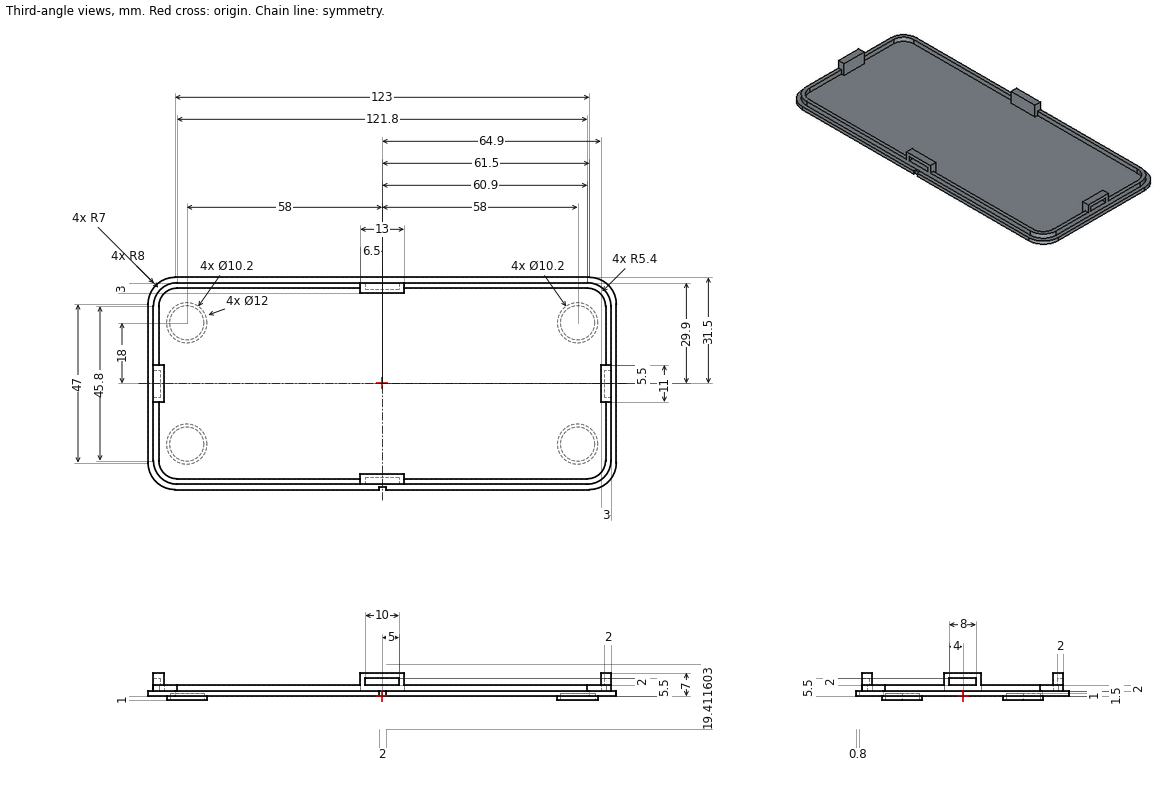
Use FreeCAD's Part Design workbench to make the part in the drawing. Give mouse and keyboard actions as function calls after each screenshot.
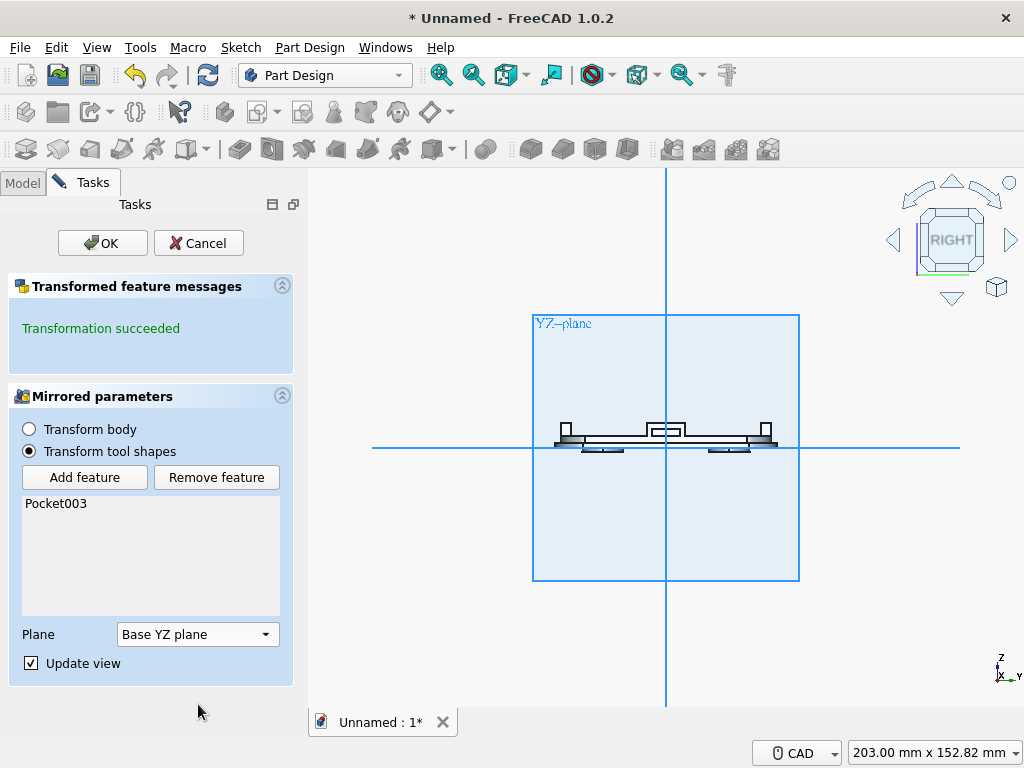
click(103, 243)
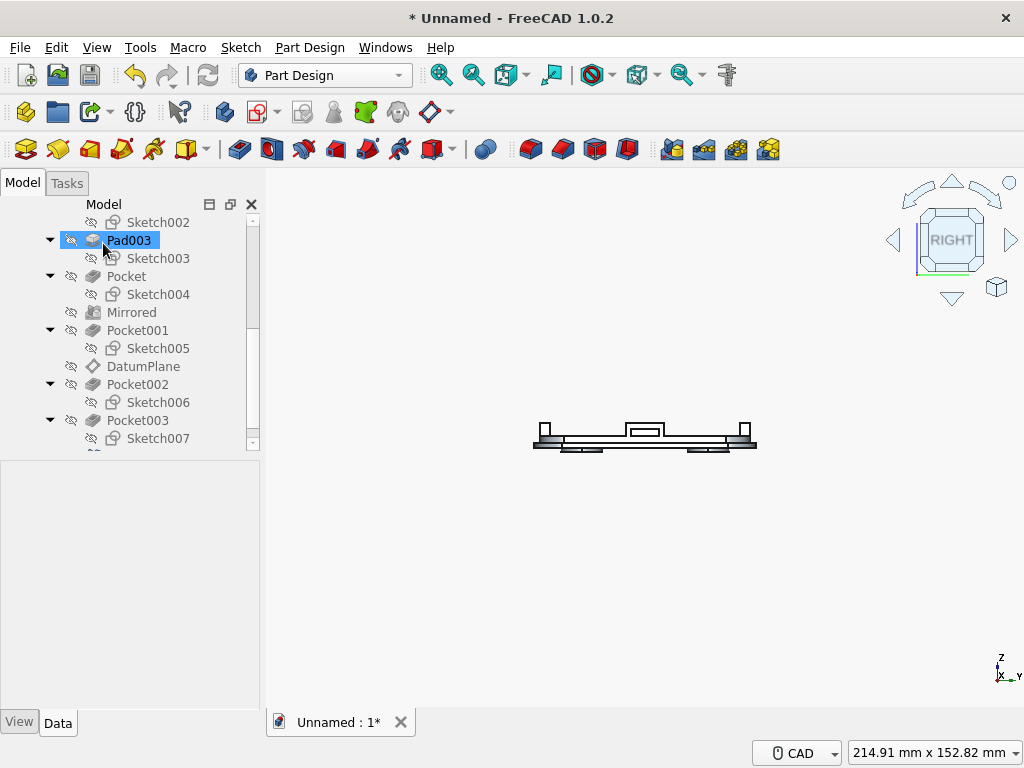
key(0)